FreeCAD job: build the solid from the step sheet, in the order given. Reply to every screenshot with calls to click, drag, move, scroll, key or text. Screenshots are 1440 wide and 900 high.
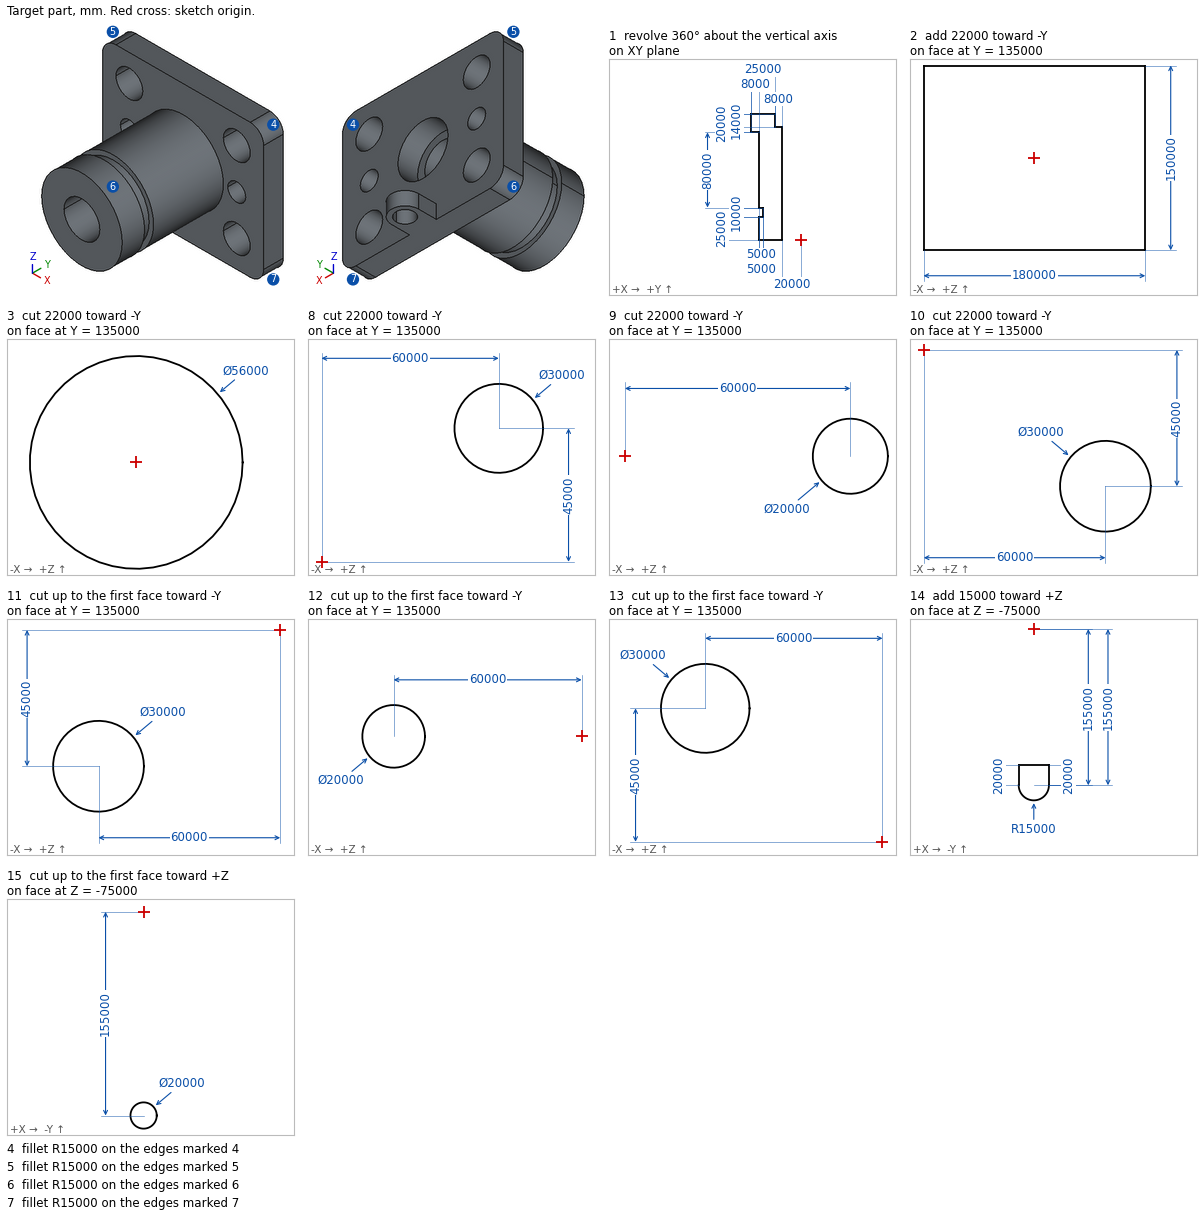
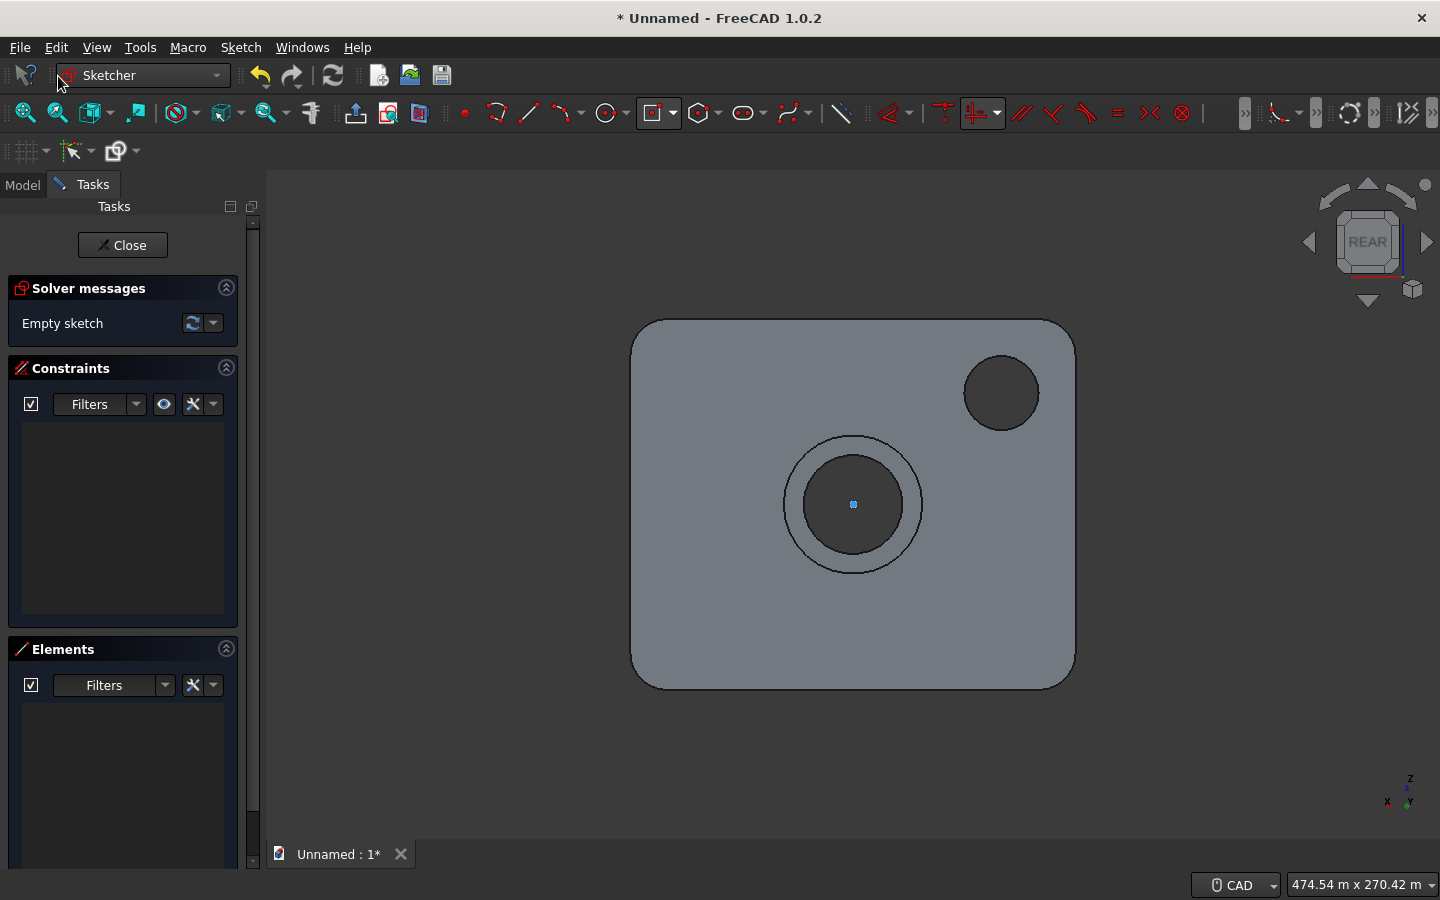
scroll(1028, 504, up, 11)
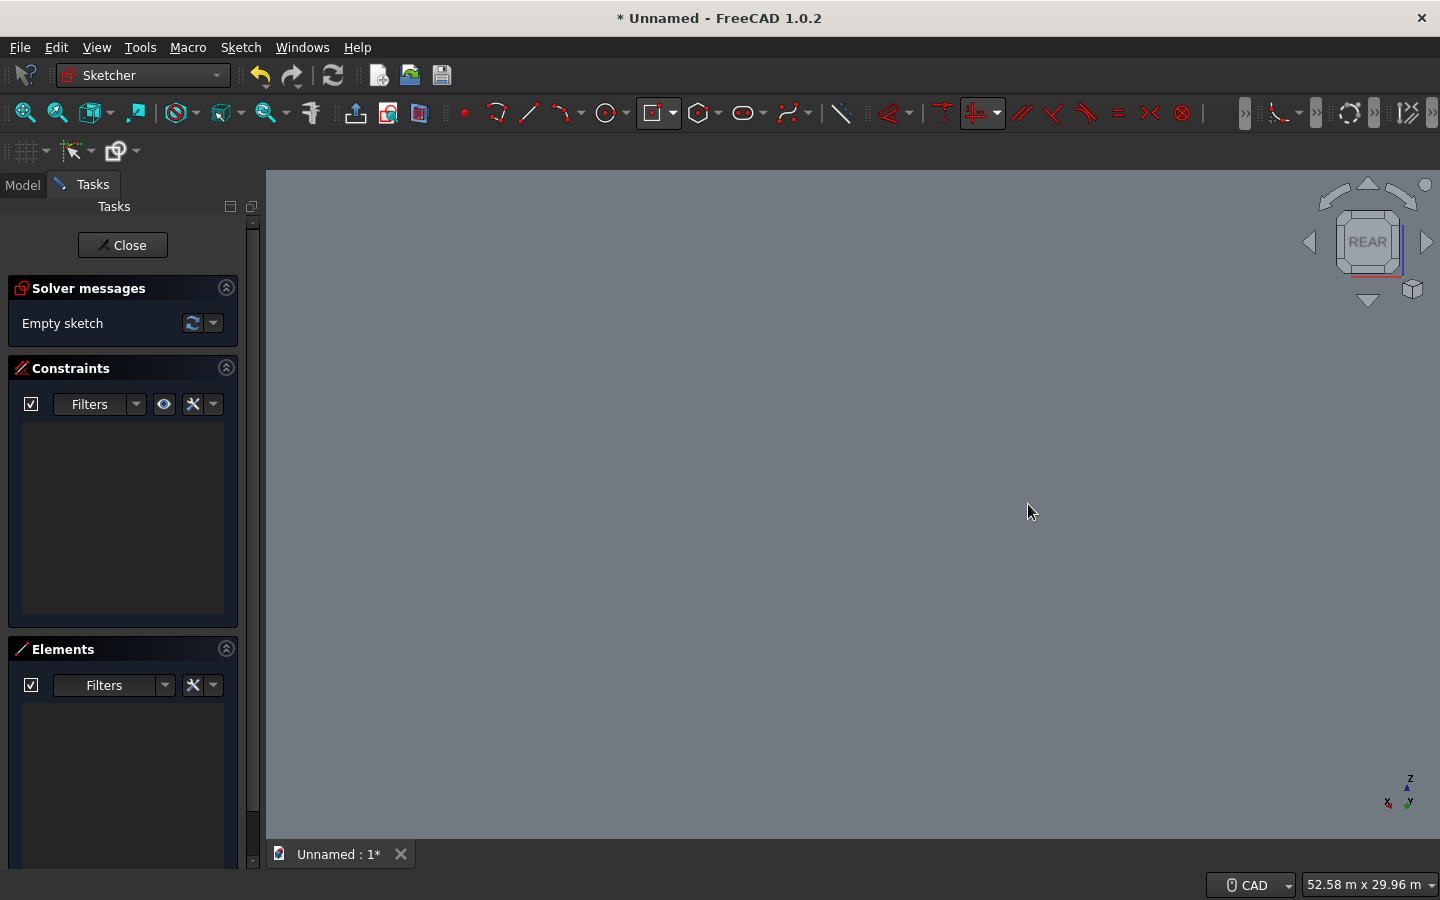
key(g)
key(c)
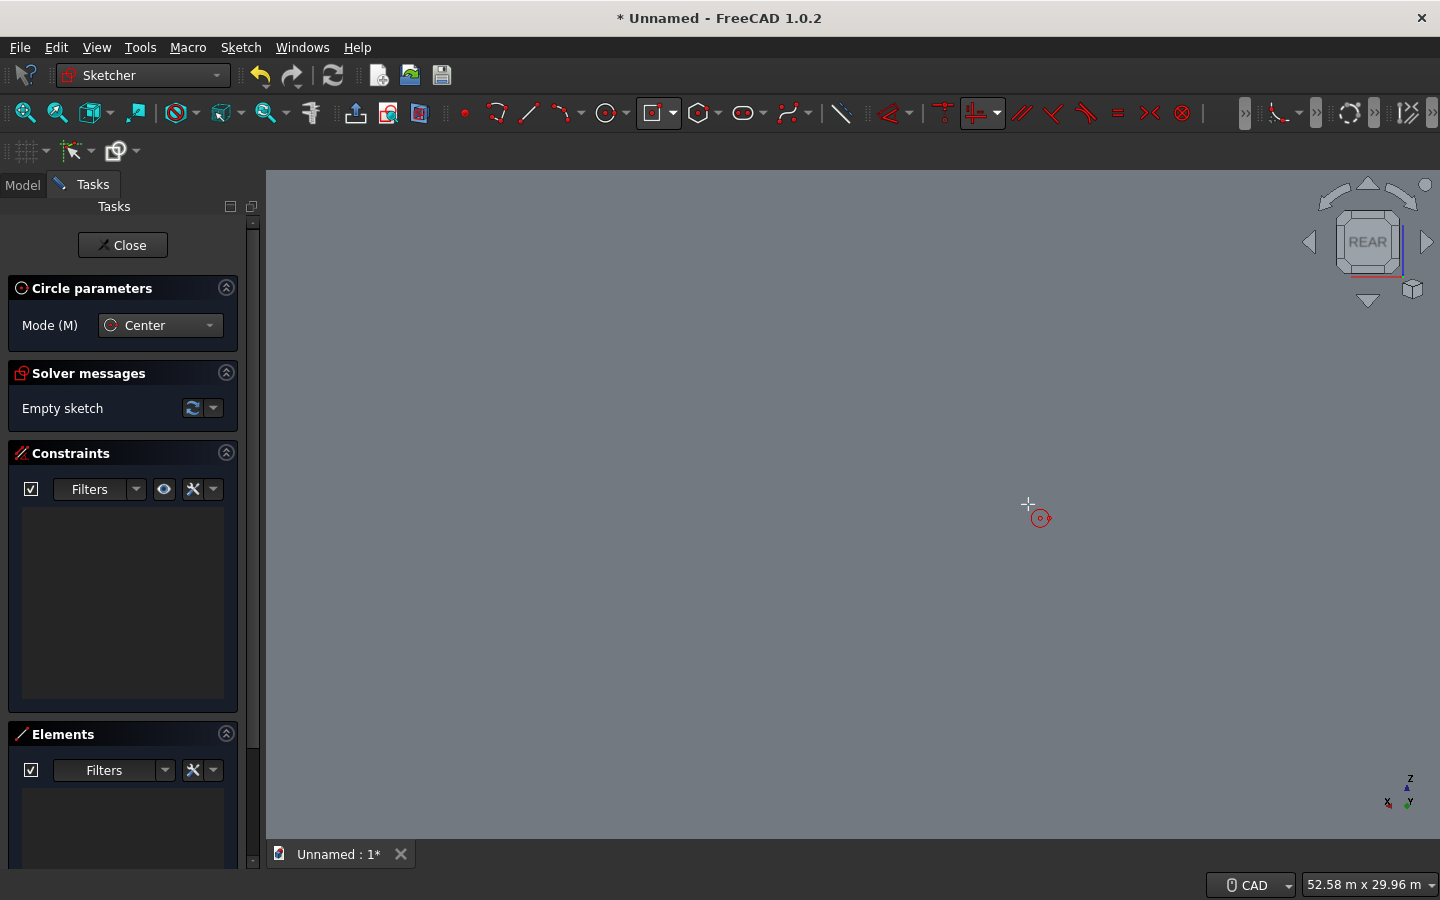
click(783, 504)
click(941, 347)
key(Escape)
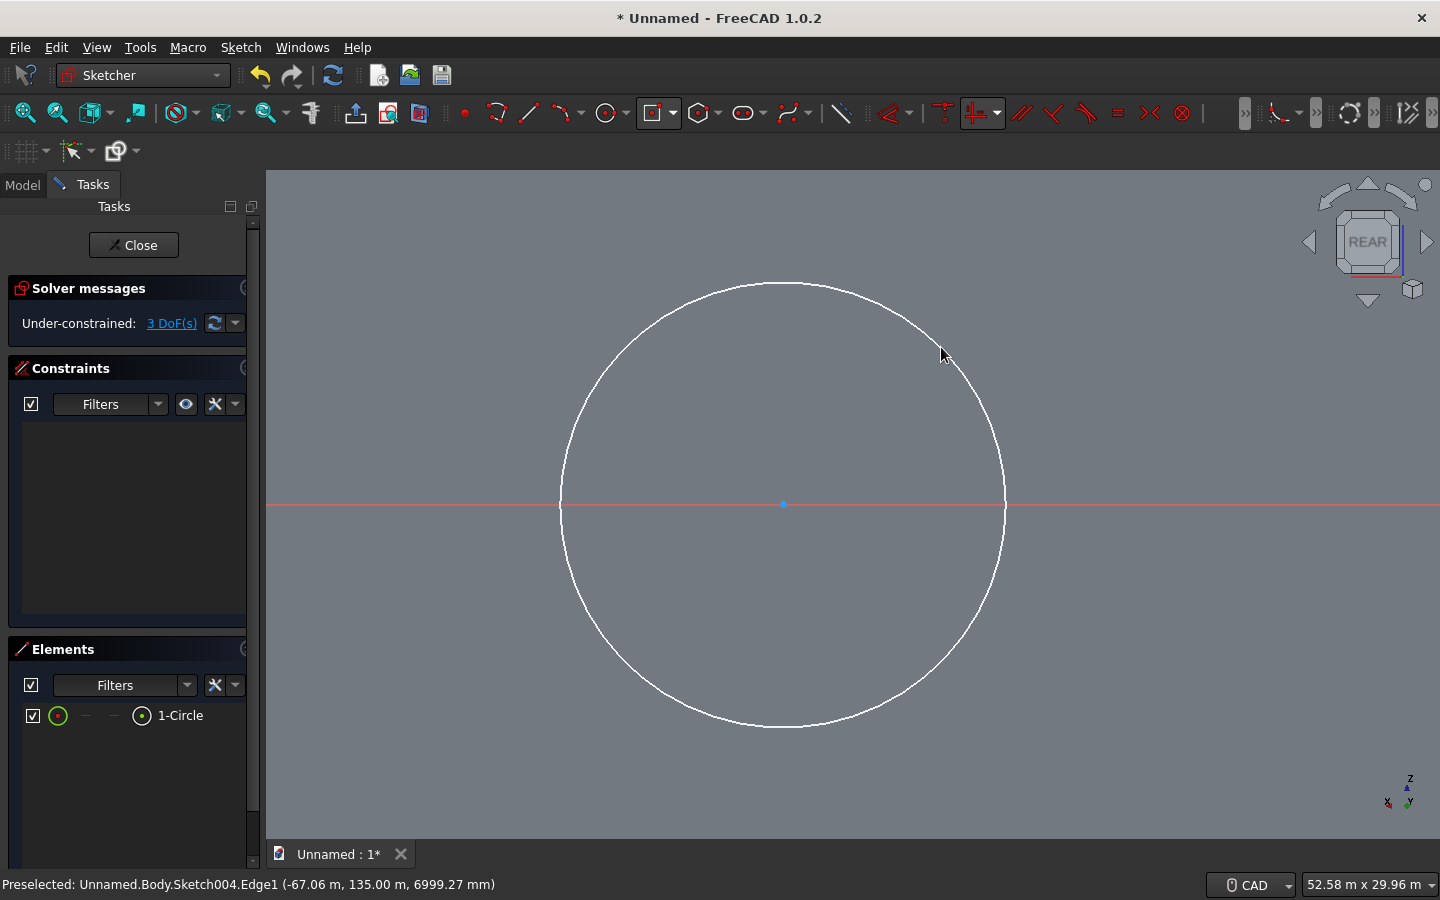
click(783, 505)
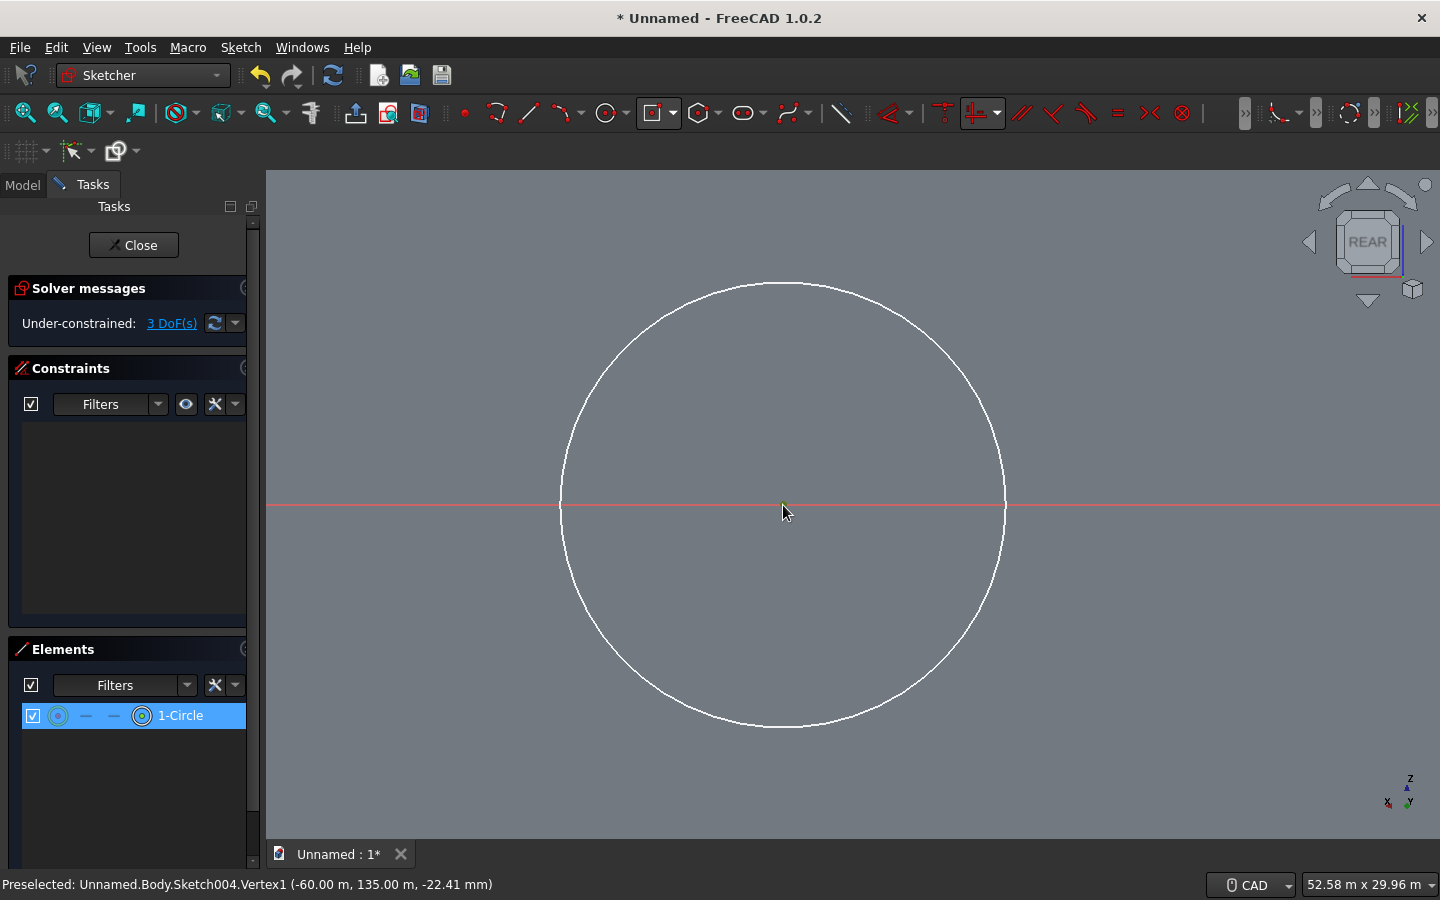
click(364, 504)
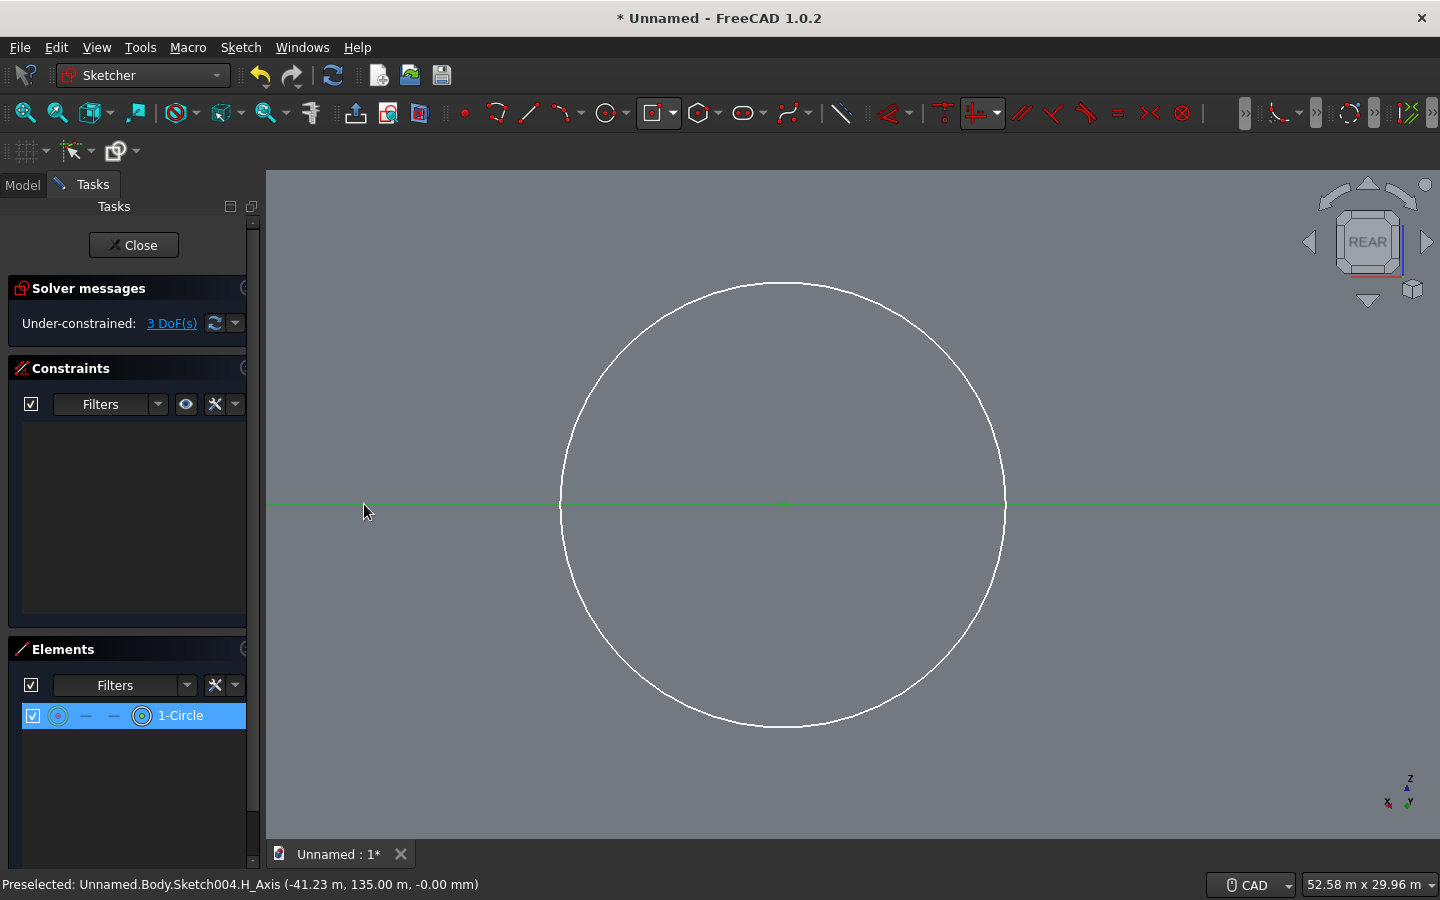
click(944, 114)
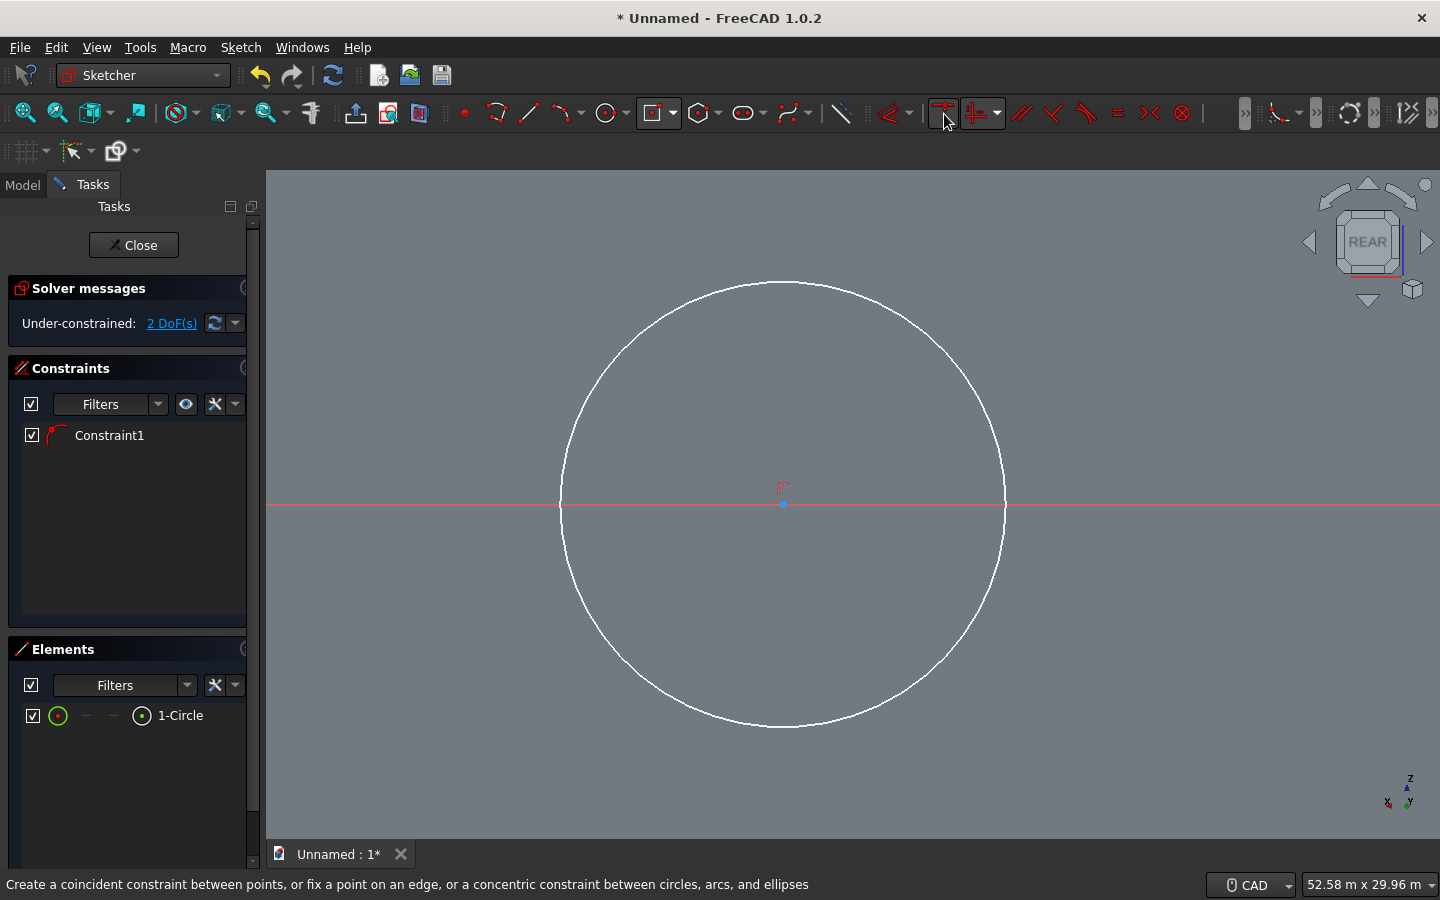
key(d)